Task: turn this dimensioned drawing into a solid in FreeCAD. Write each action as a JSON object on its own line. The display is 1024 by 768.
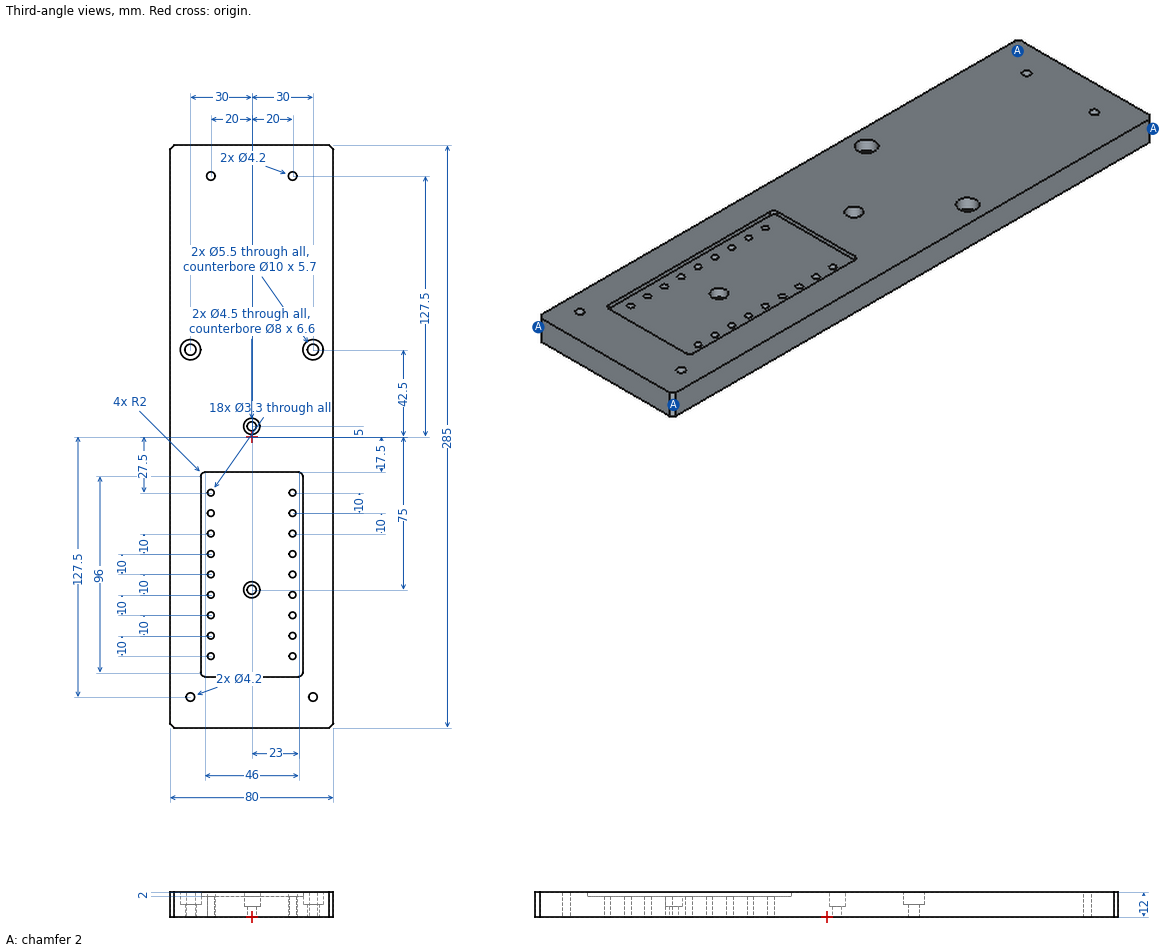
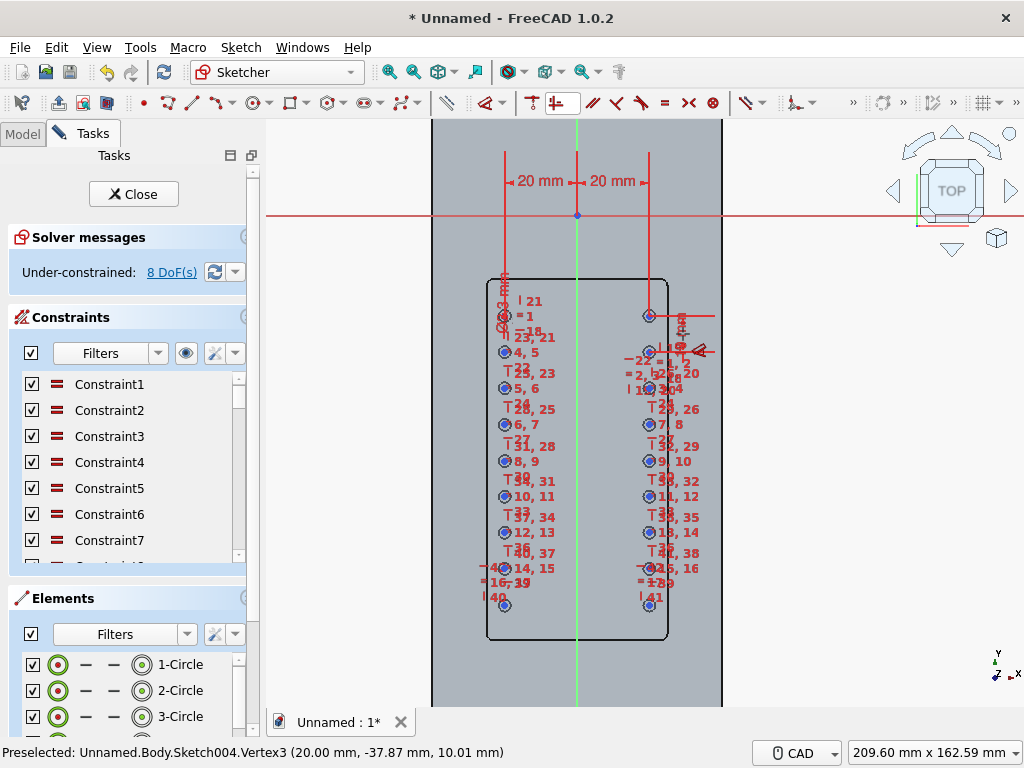
{"action": "left_click", "coordinate": [649, 352]}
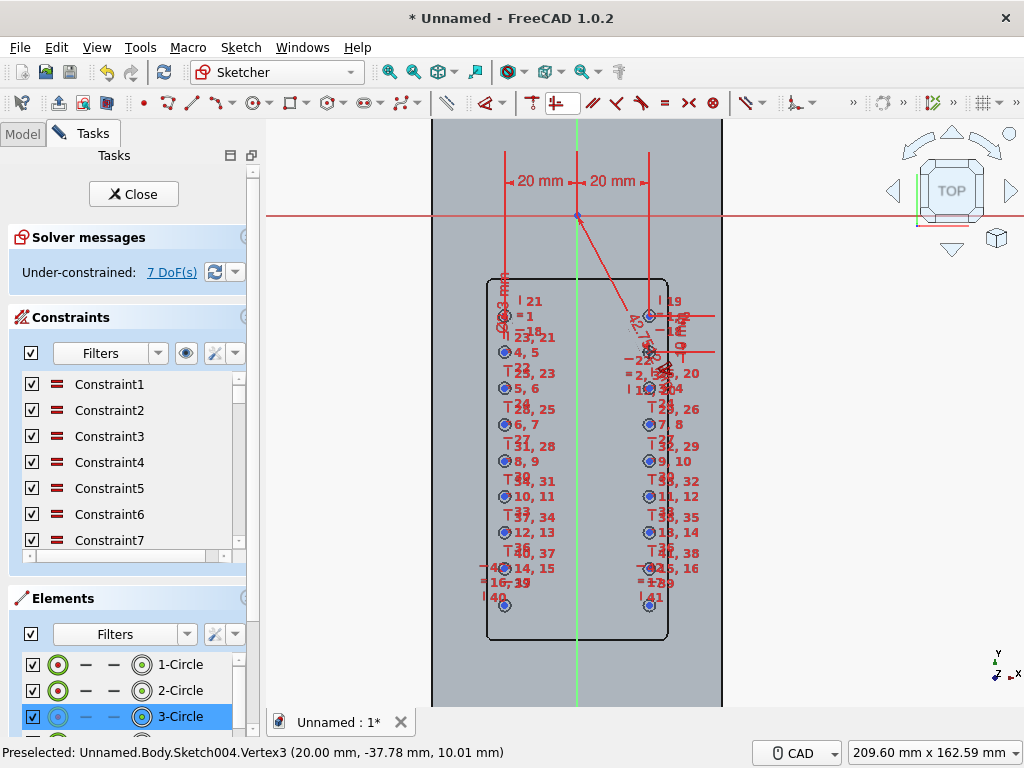
{"action": "left_click", "coordinate": [649, 388]}
{"action": "left_click", "coordinate": [683, 370]}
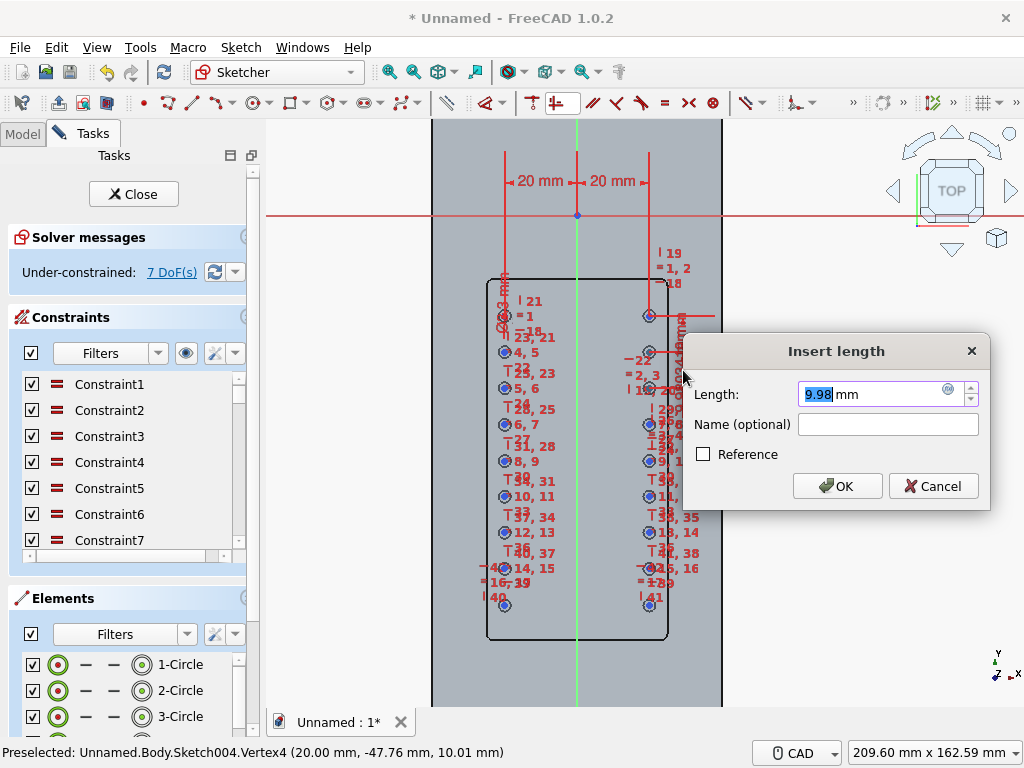
{"action": "type", "text": "10"}
{"action": "key", "text": "Return"}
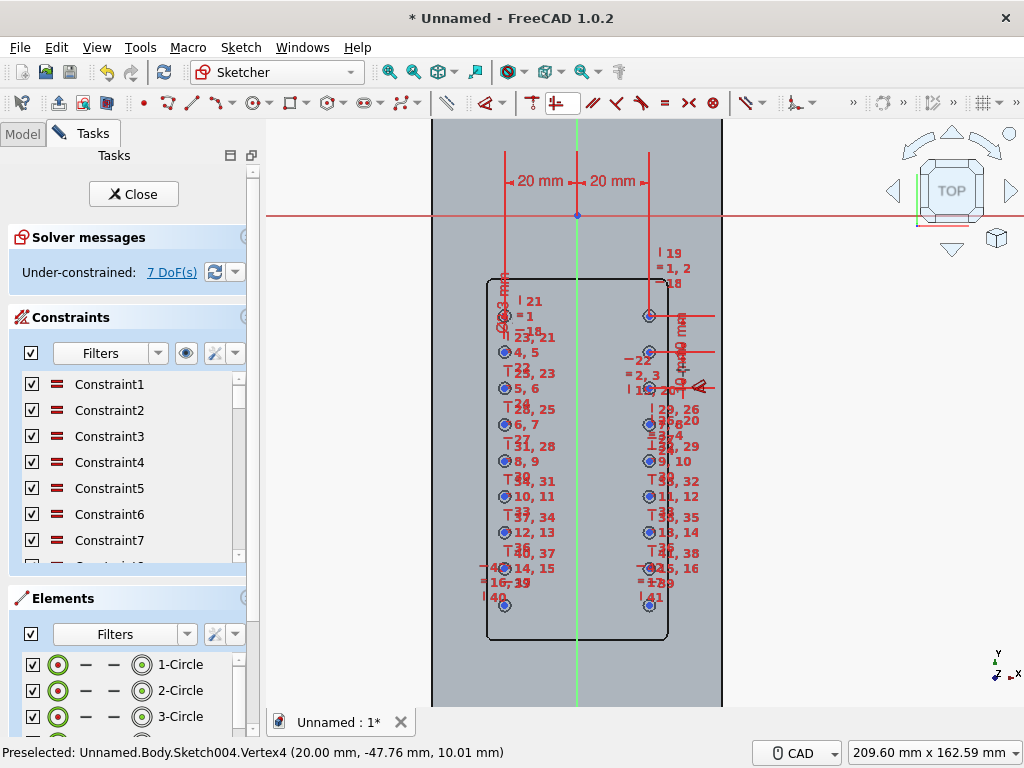
{"action": "left_click", "coordinate": [505, 388]}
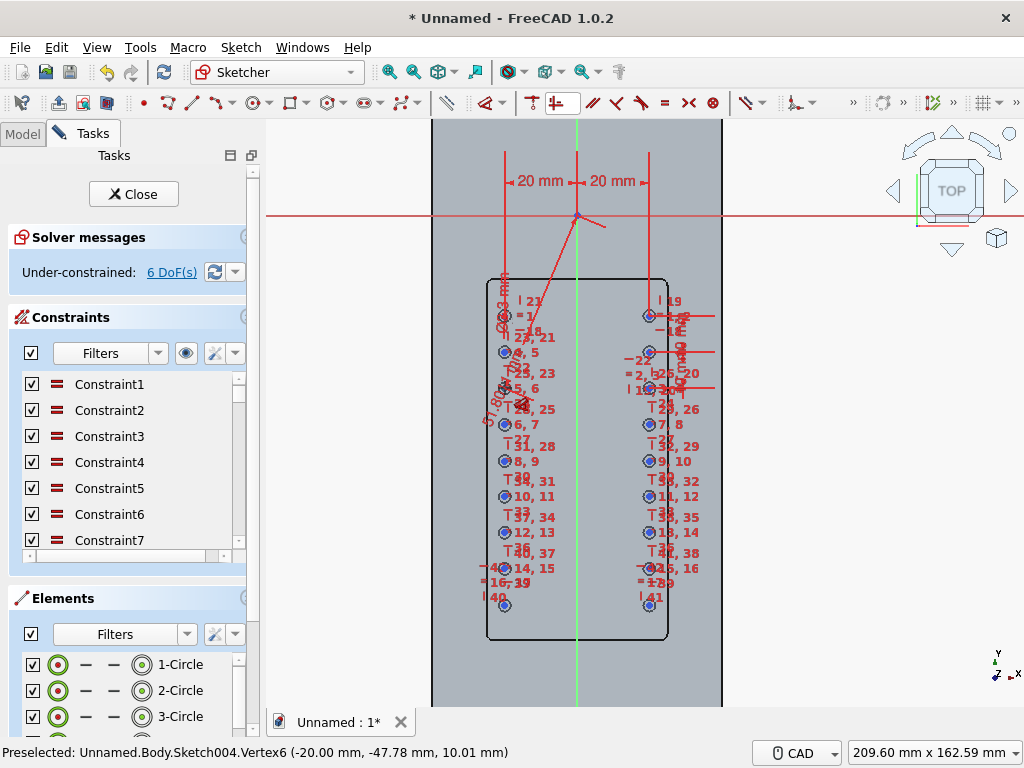
{"action": "left_click", "coordinate": [505, 425]}
{"action": "left_click", "coordinate": [471, 407]}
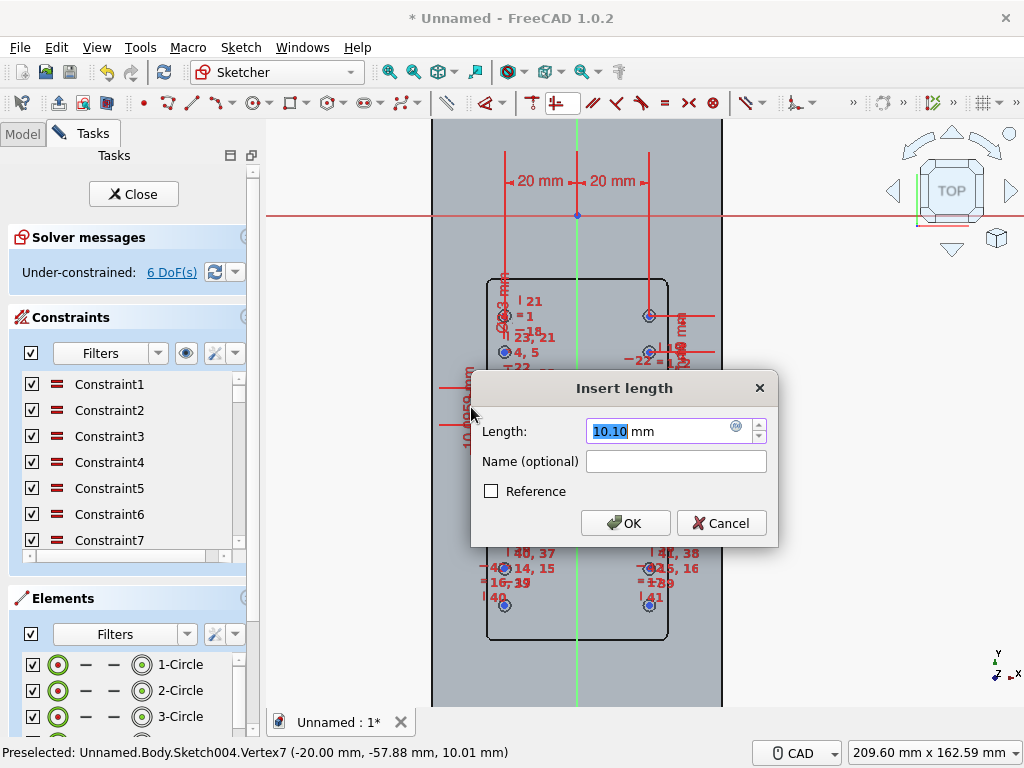
{"action": "type", "text": "10"}
{"action": "key", "text": "Return"}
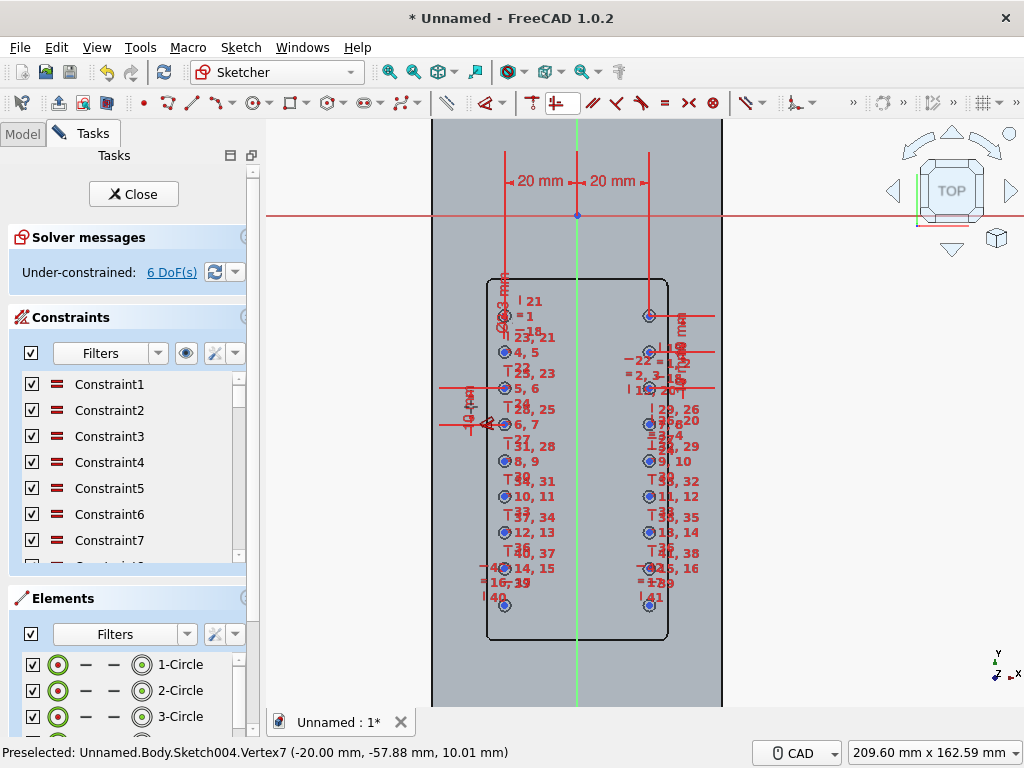
{"action": "left_click", "coordinate": [505, 425]}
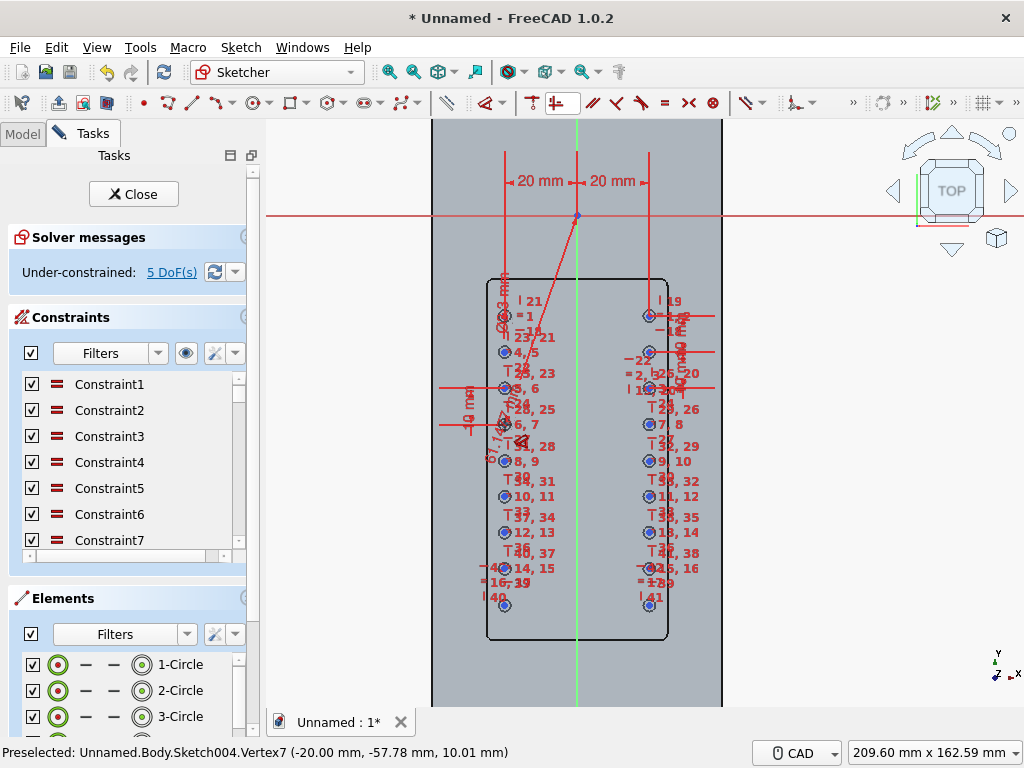
{"action": "left_click", "coordinate": [505, 461]}
{"action": "left_click", "coordinate": [471, 443]}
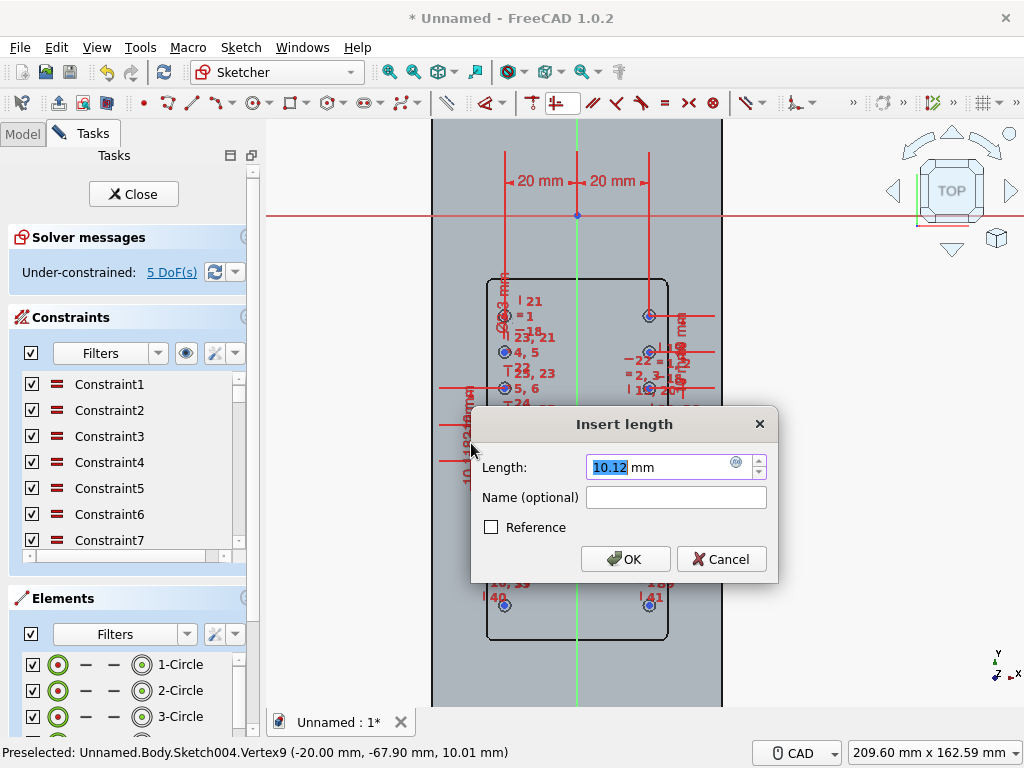
{"action": "type", "text": "10"}
{"action": "key", "text": "Return"}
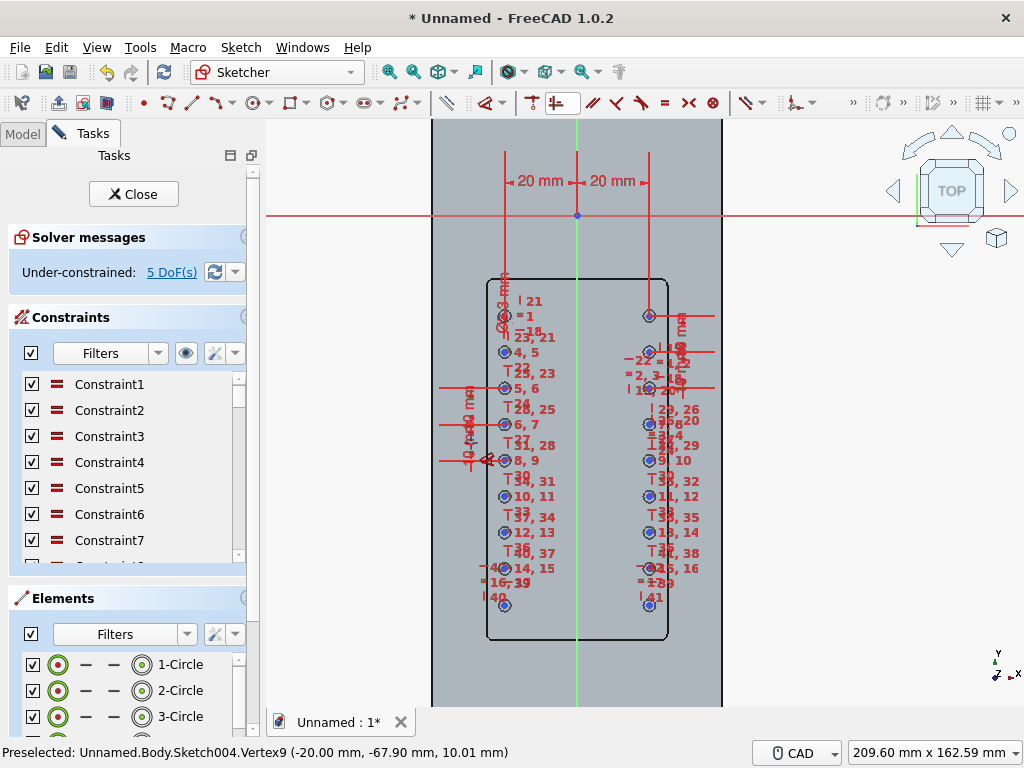
{"action": "left_click", "coordinate": [505, 461]}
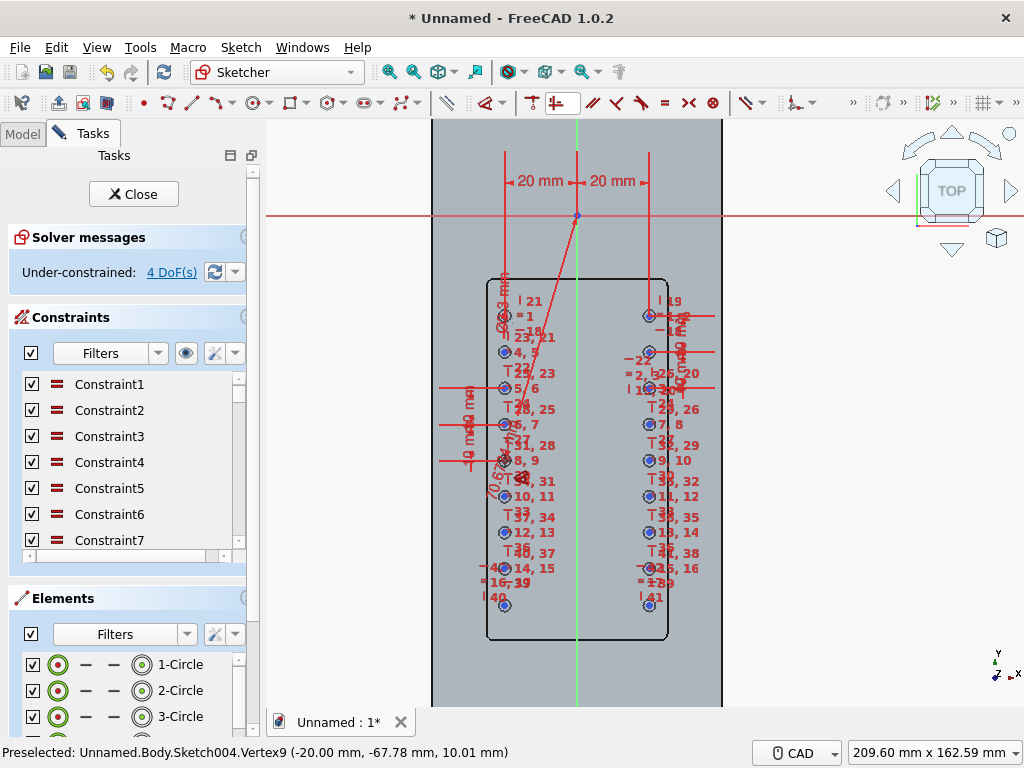
{"action": "left_click", "coordinate": [505, 497]}
{"action": "left_click", "coordinate": [471, 479]}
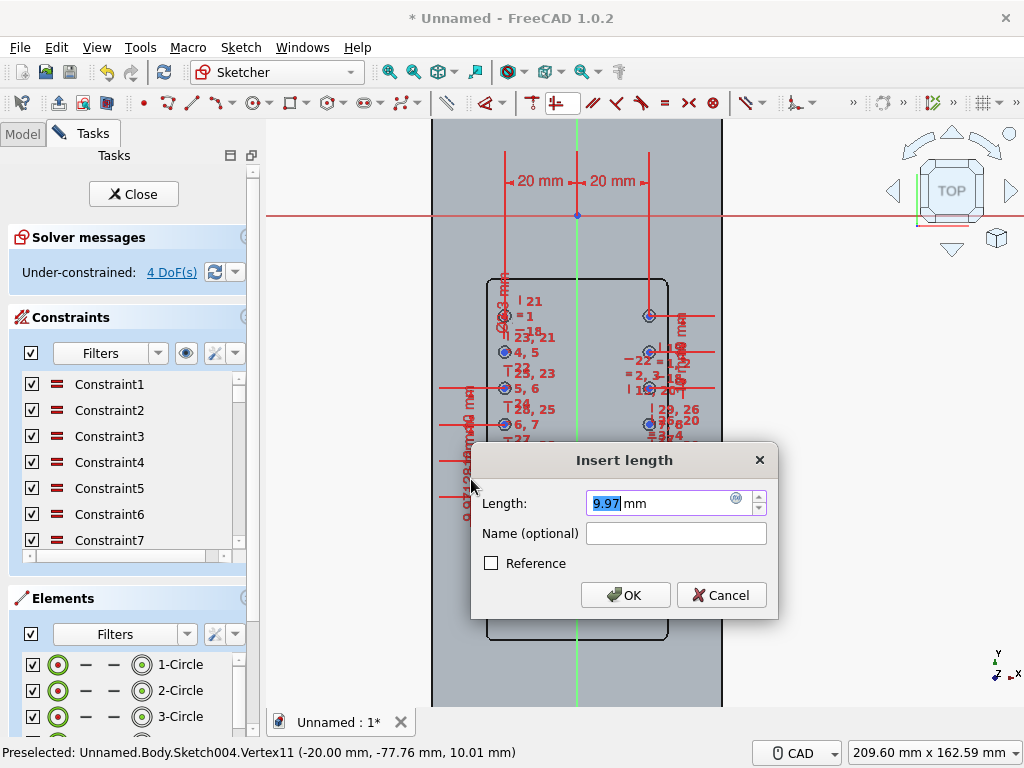
{"action": "type", "text": "10"}
{"action": "key", "text": "Return"}